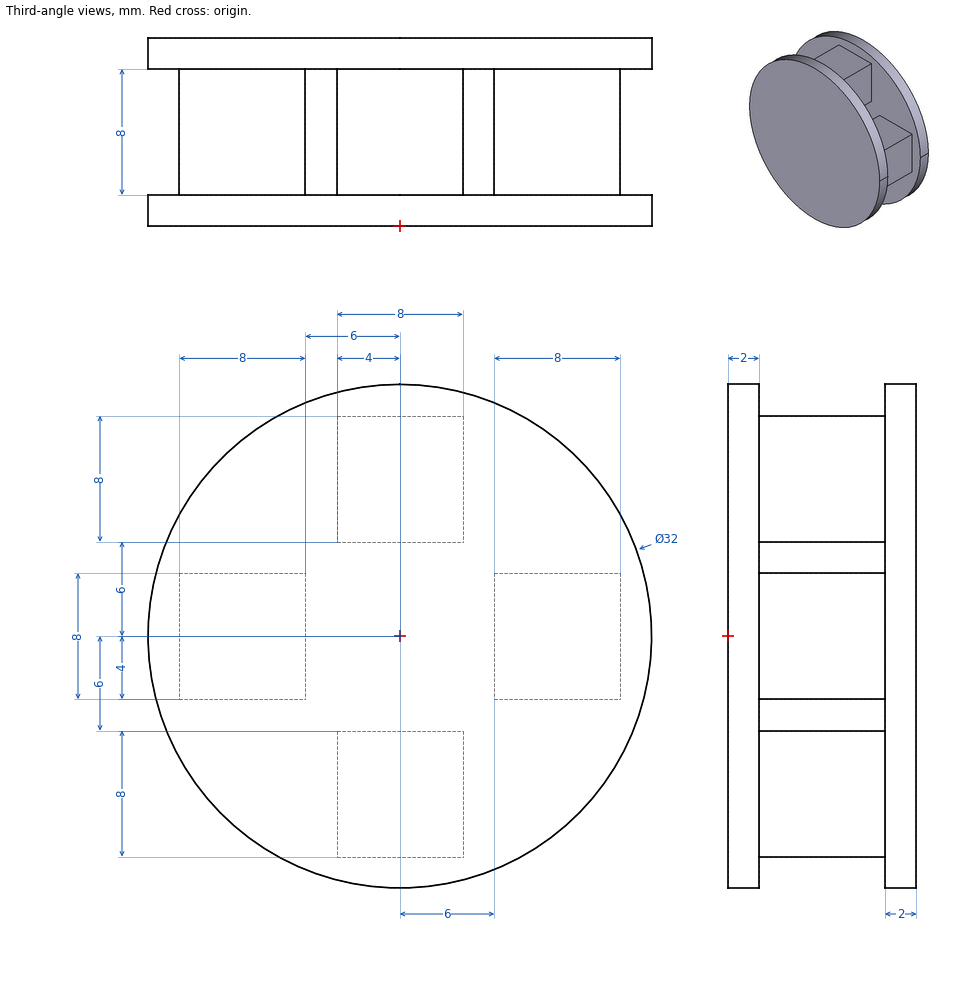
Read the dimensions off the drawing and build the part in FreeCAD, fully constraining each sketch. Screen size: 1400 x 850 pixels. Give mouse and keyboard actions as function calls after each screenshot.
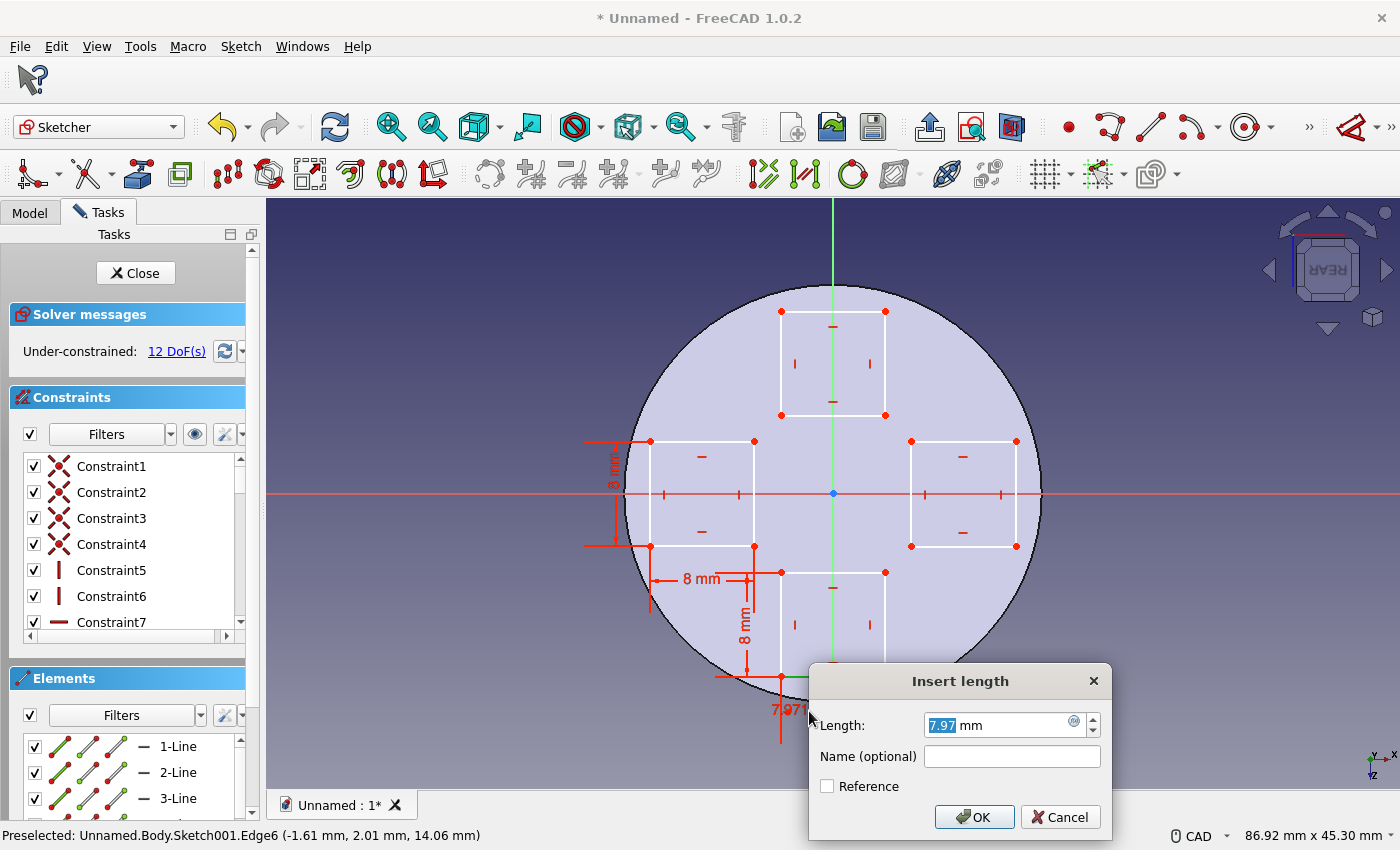
text(8)
key(Return)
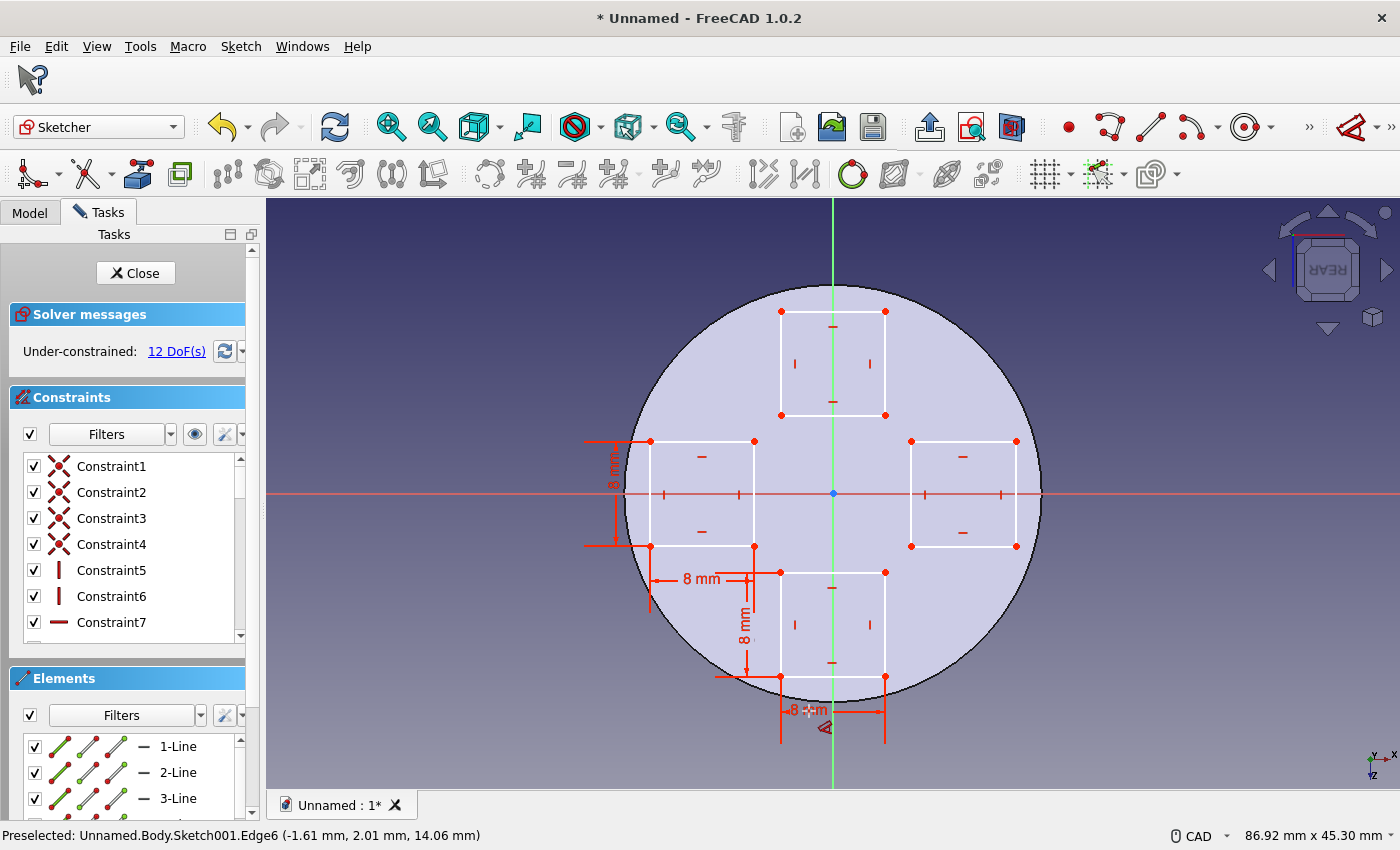
click(781, 343)
click(747, 364)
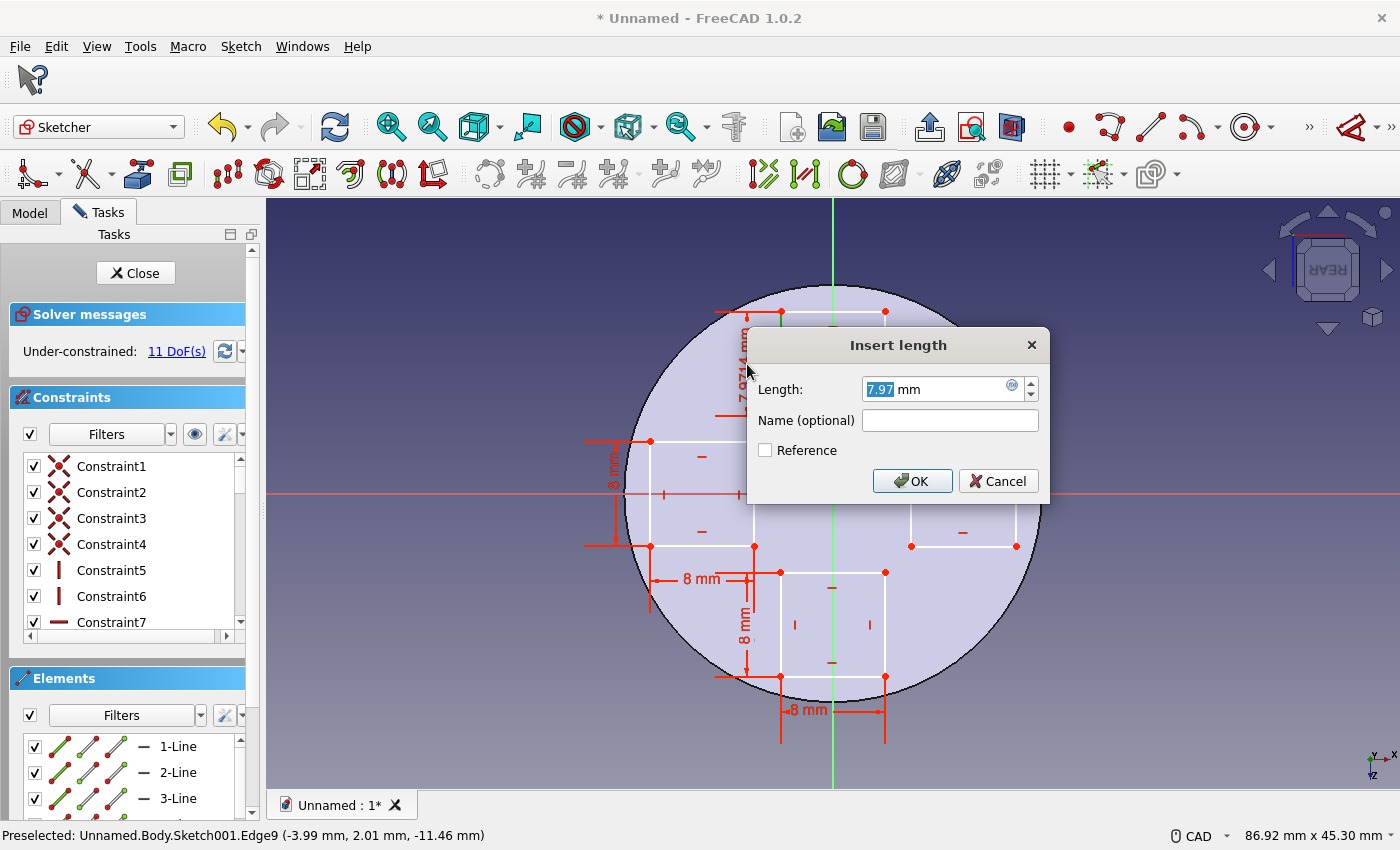
text(8)
key(Return)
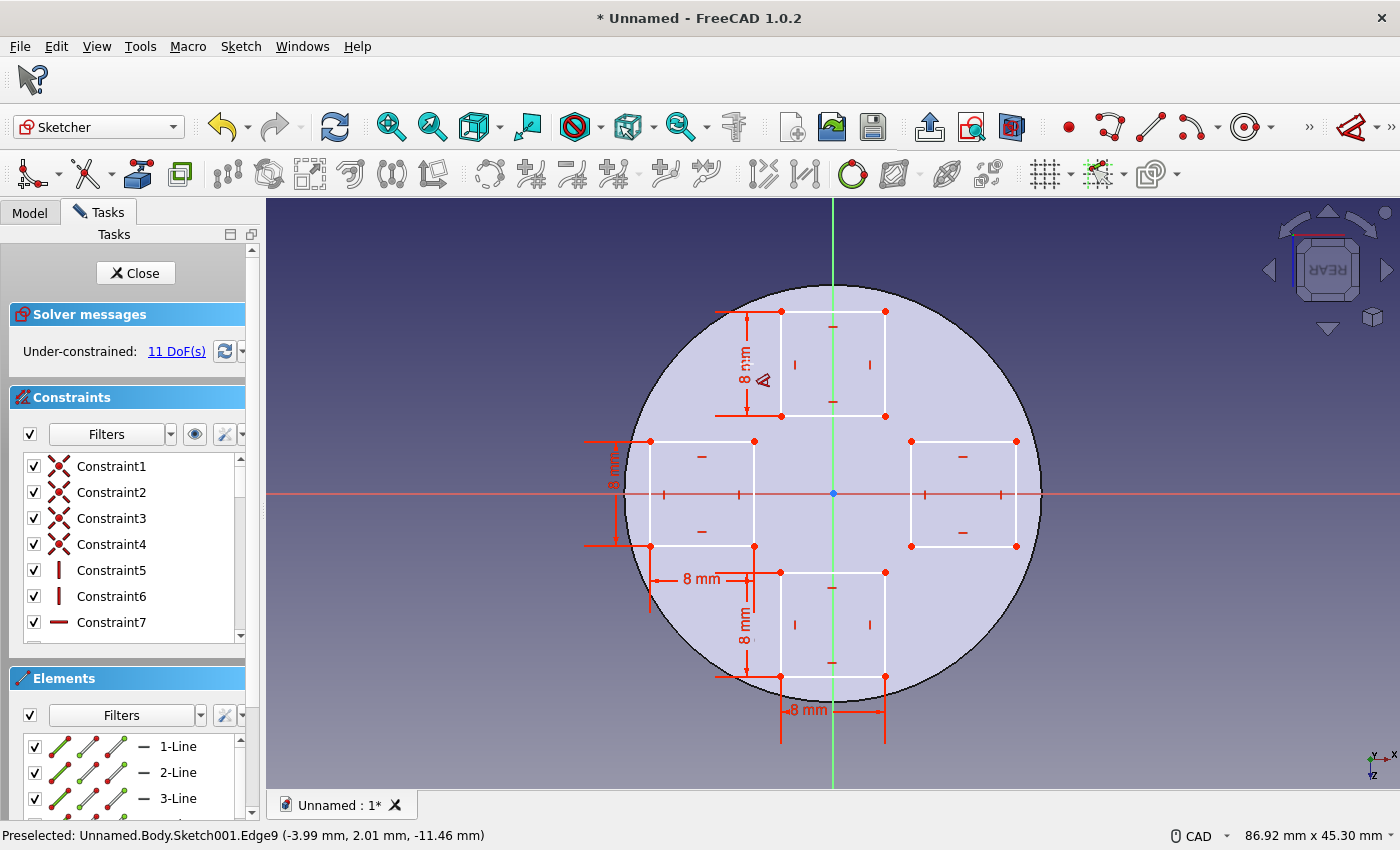
click(812, 416)
click(857, 382)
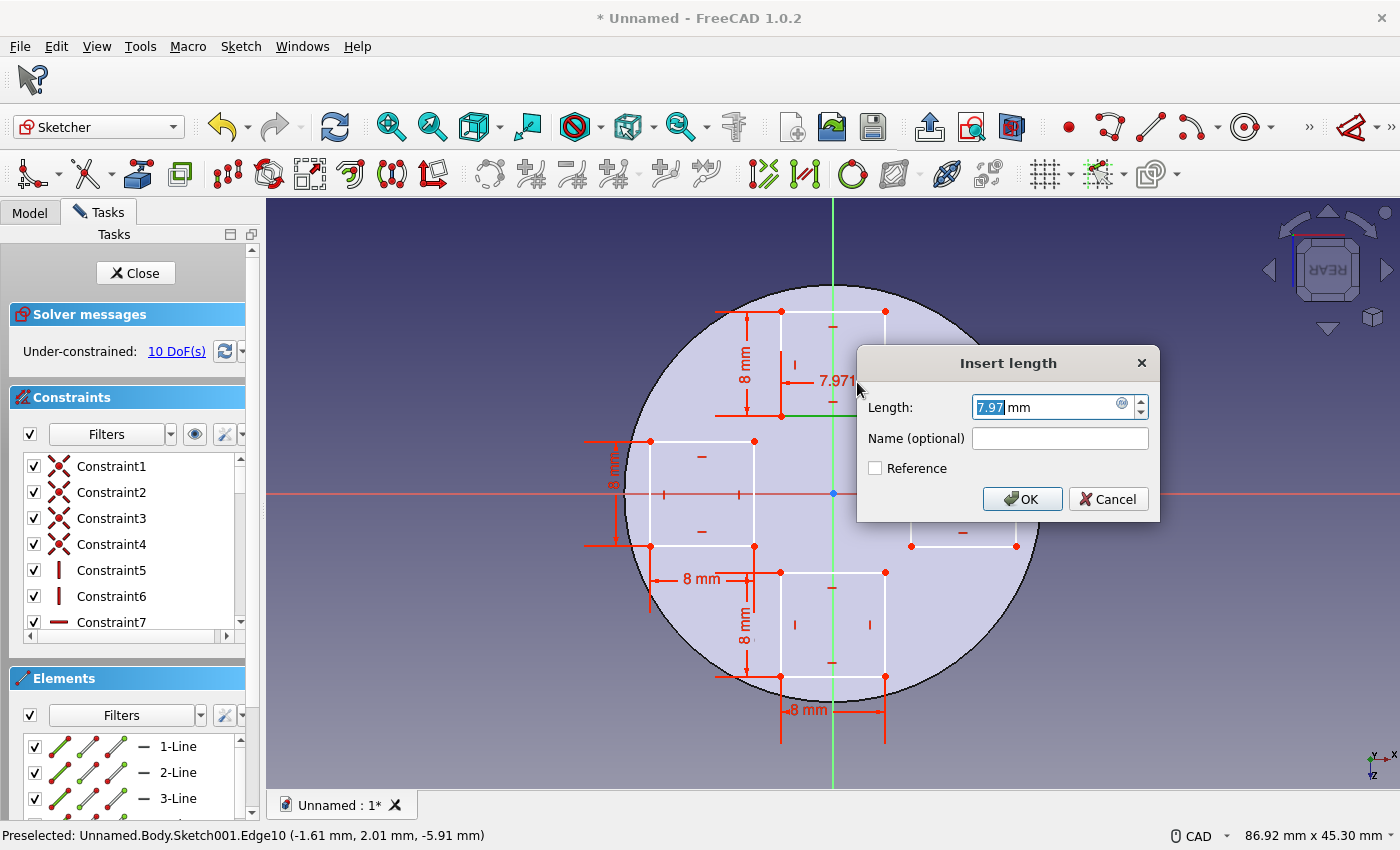
text(8)
key(Return)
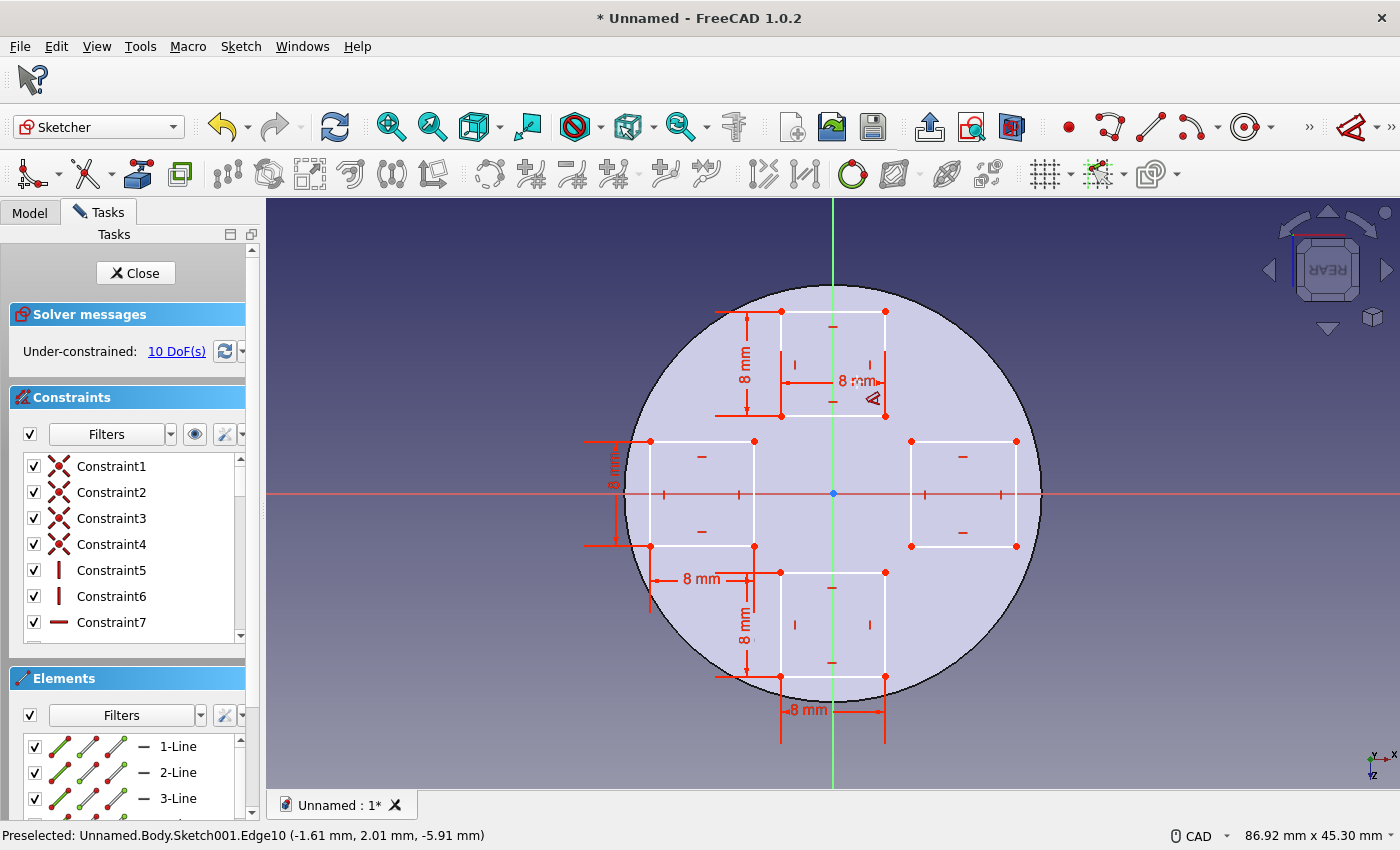
click(911, 473)
click(945, 470)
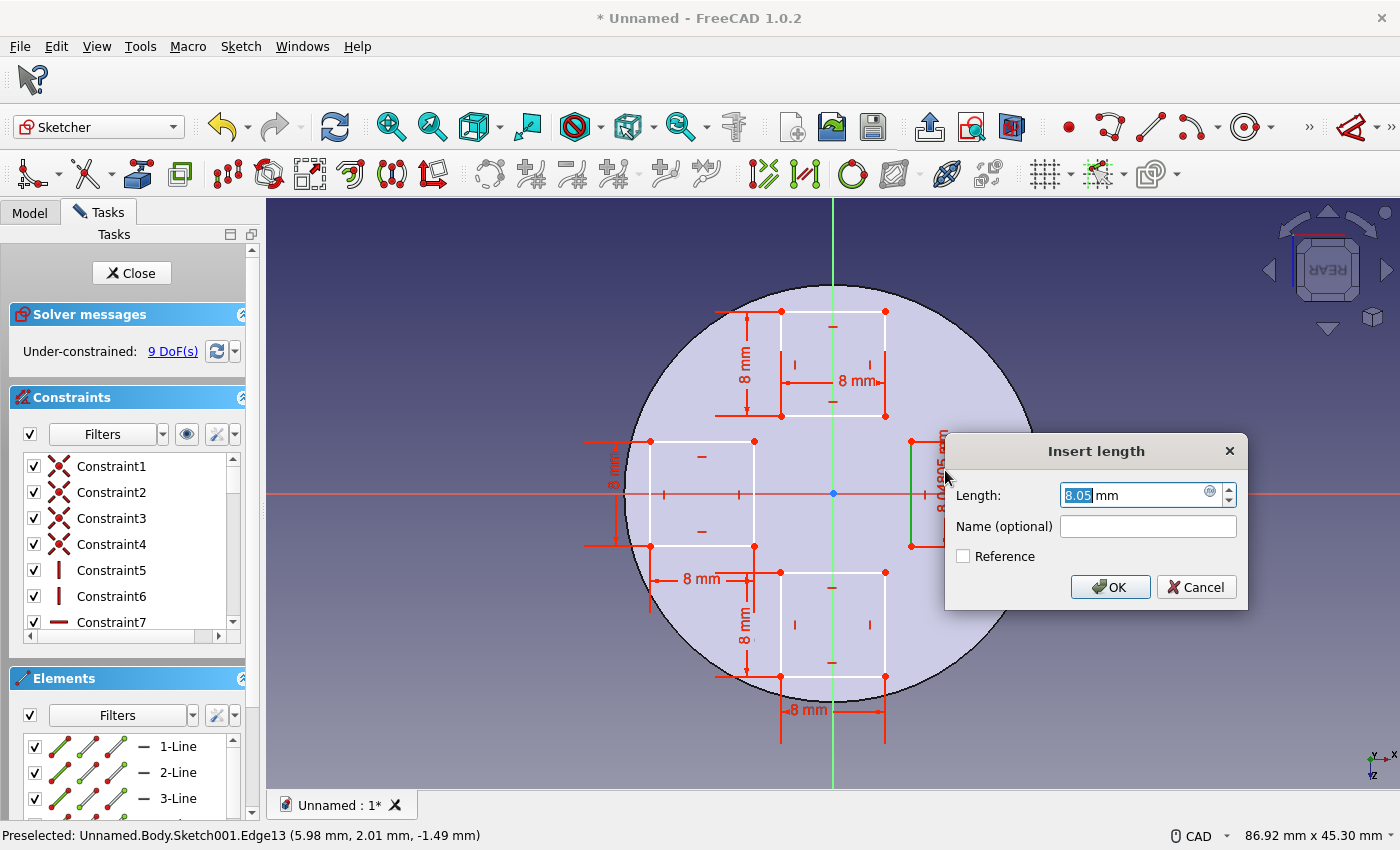
text(8)
key(Return)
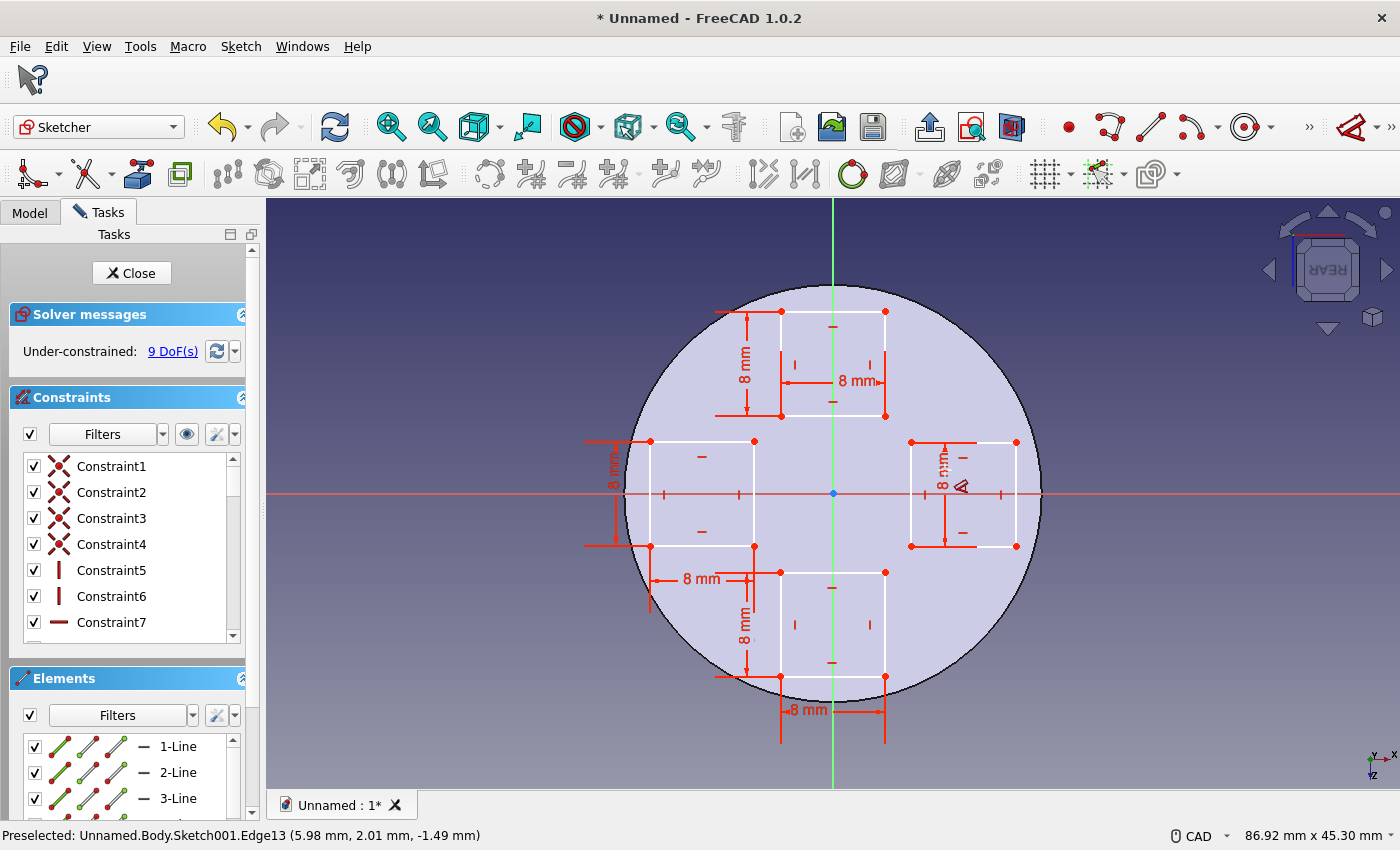
click(942, 547)
click(963, 581)